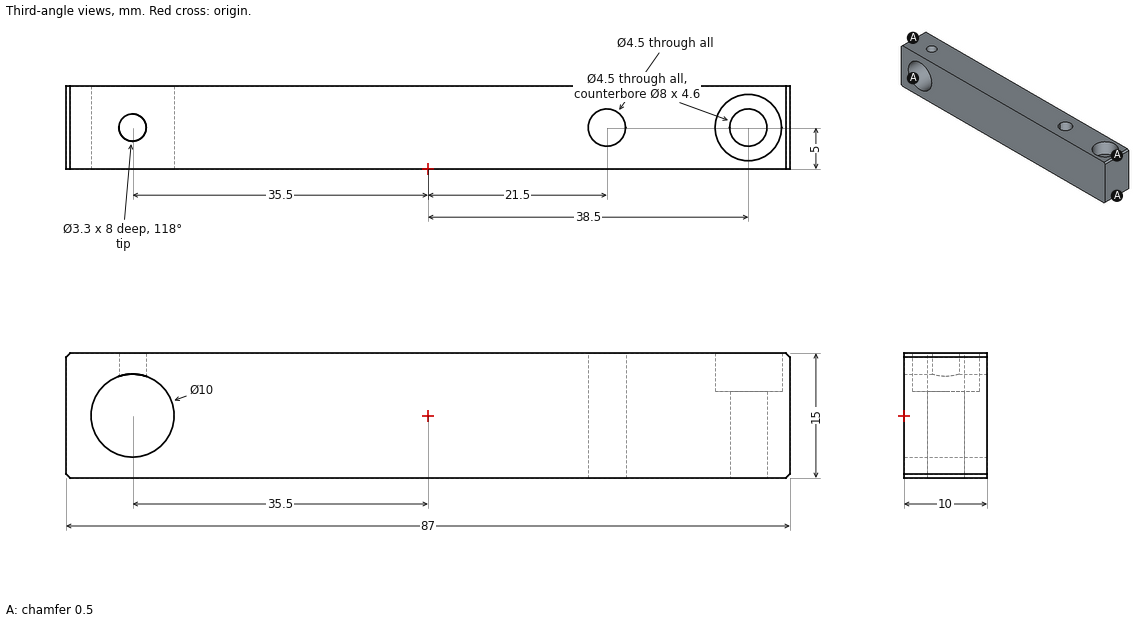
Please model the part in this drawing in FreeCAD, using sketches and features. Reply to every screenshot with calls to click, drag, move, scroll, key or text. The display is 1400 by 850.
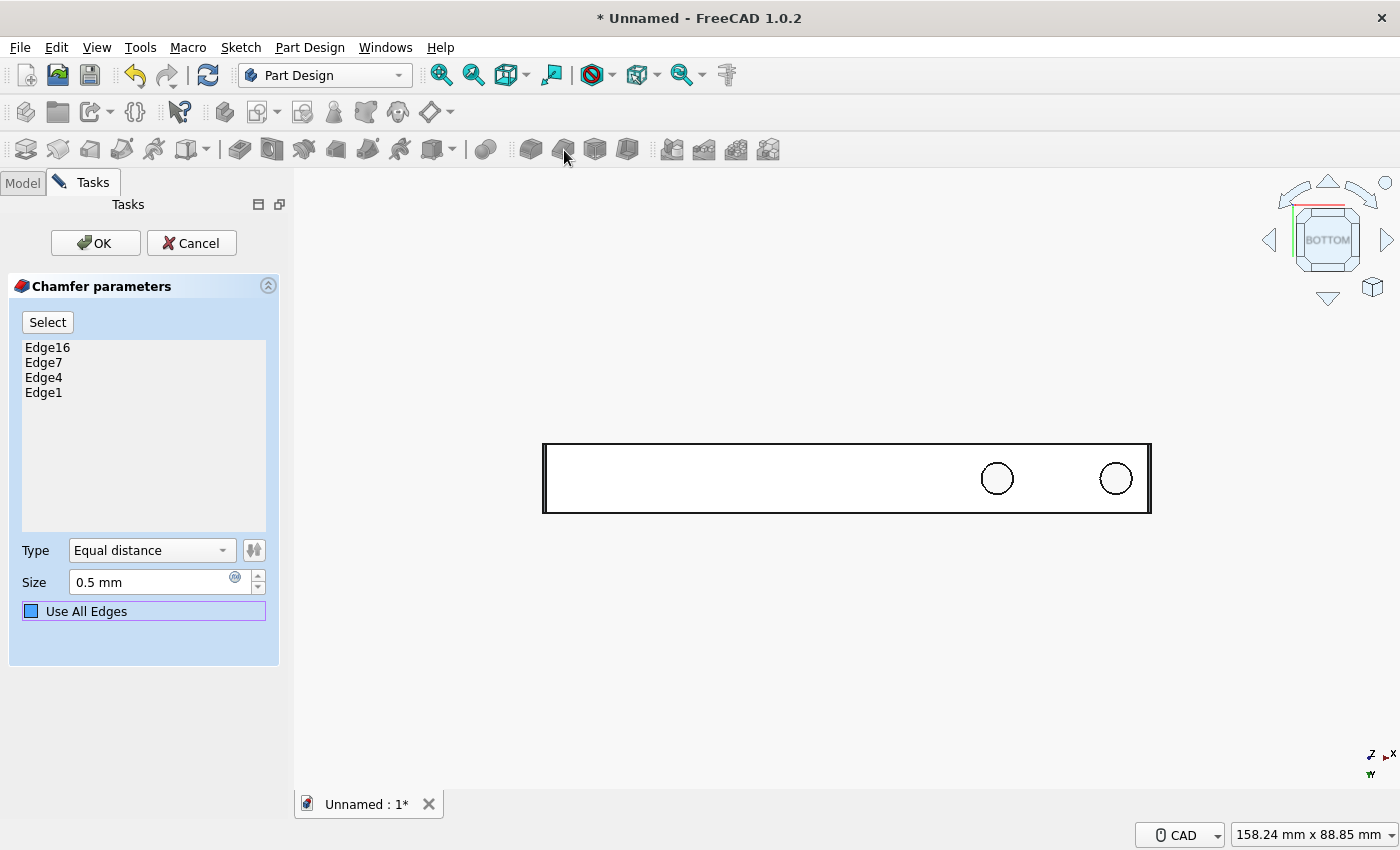
click(96, 243)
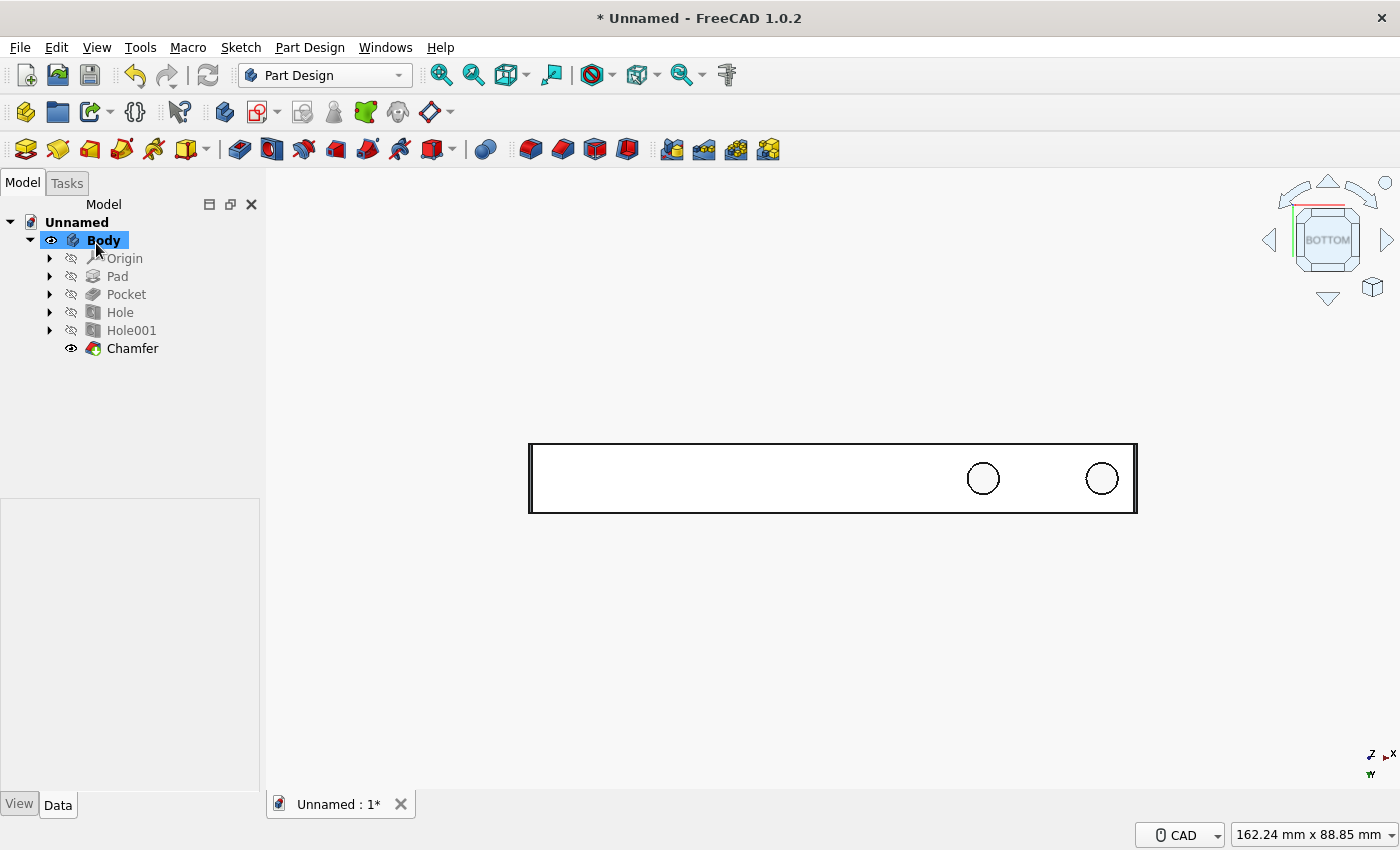
key(0)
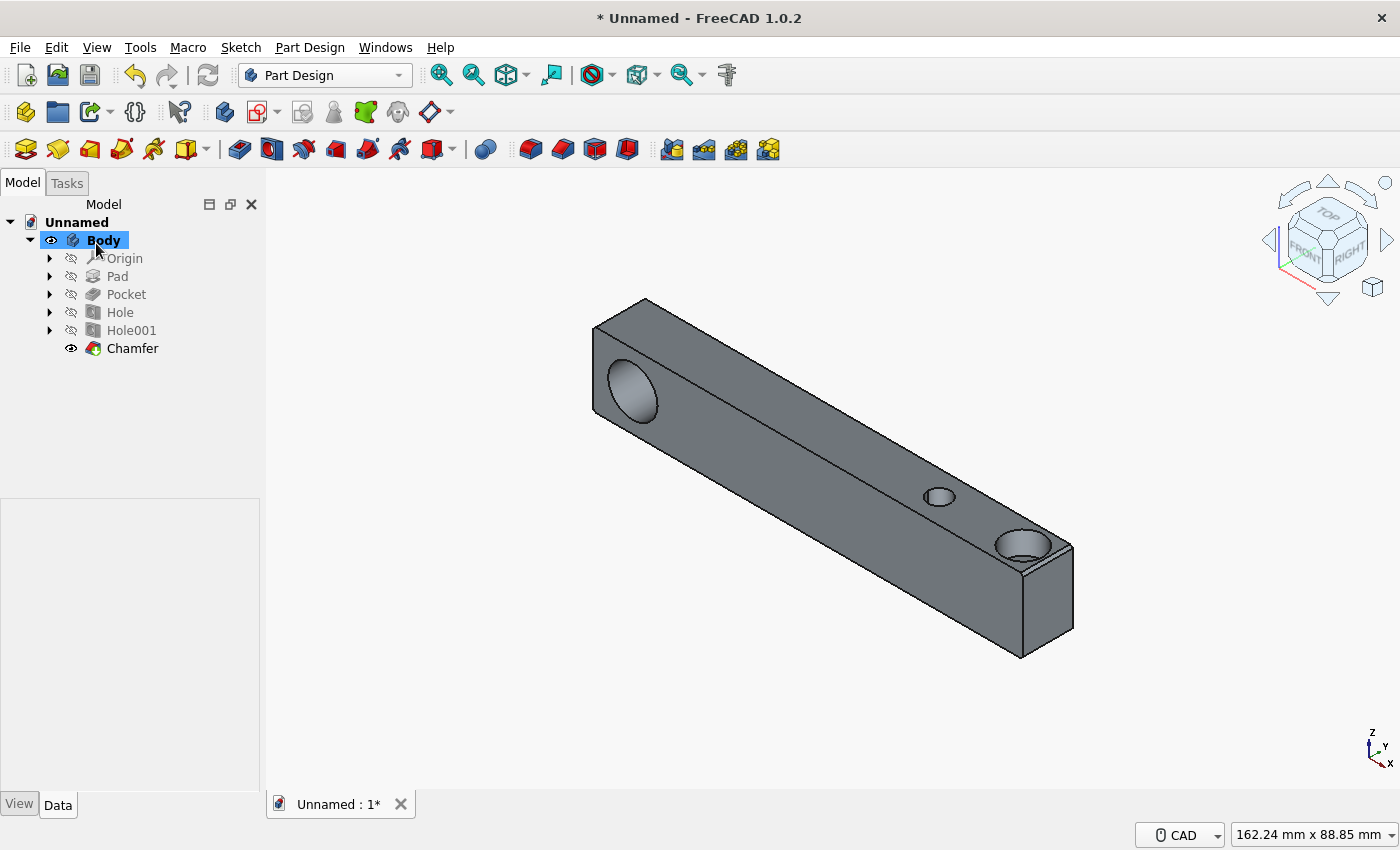
click(894, 470)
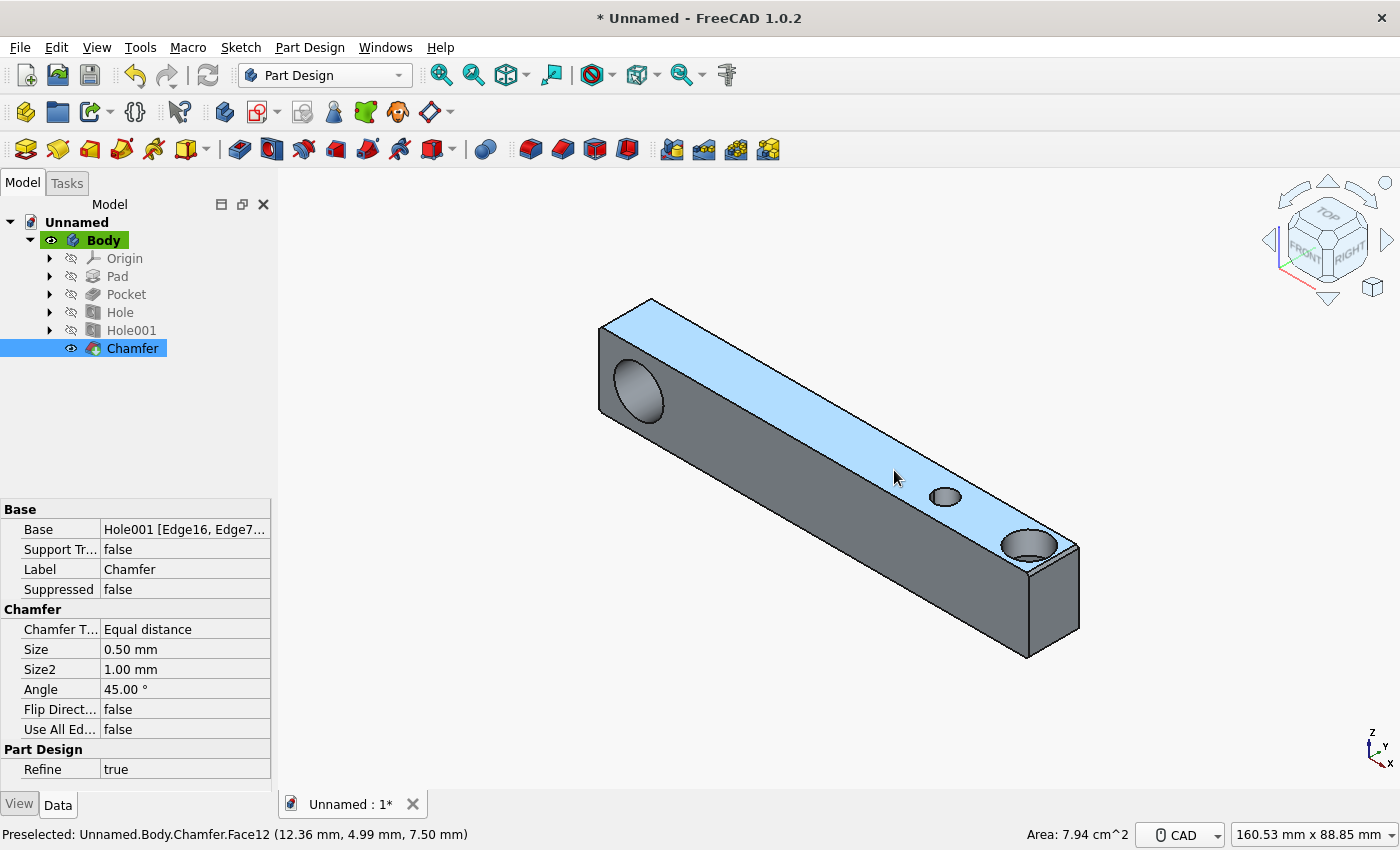
click(258, 112)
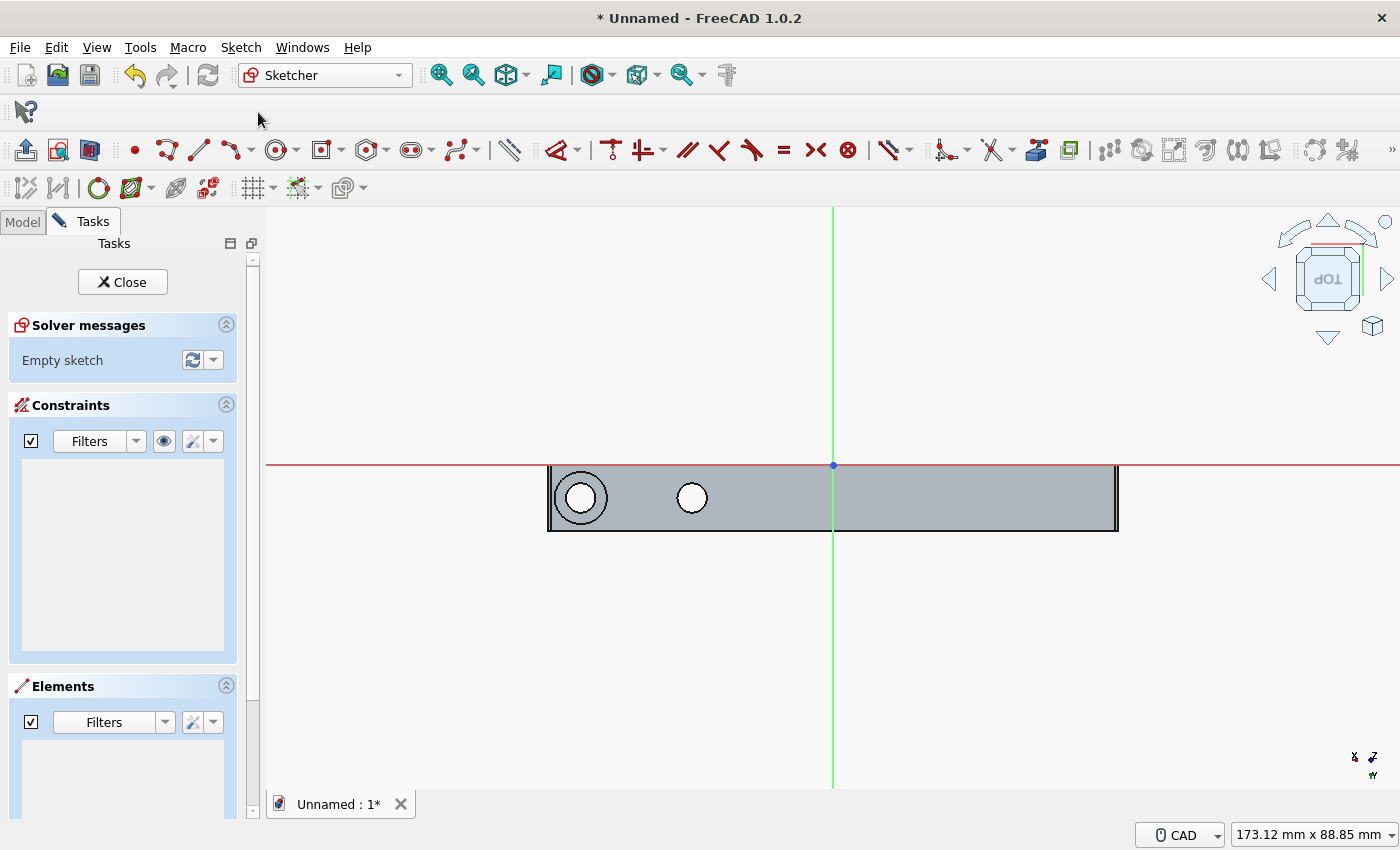
scroll(1085, 498, up, 14)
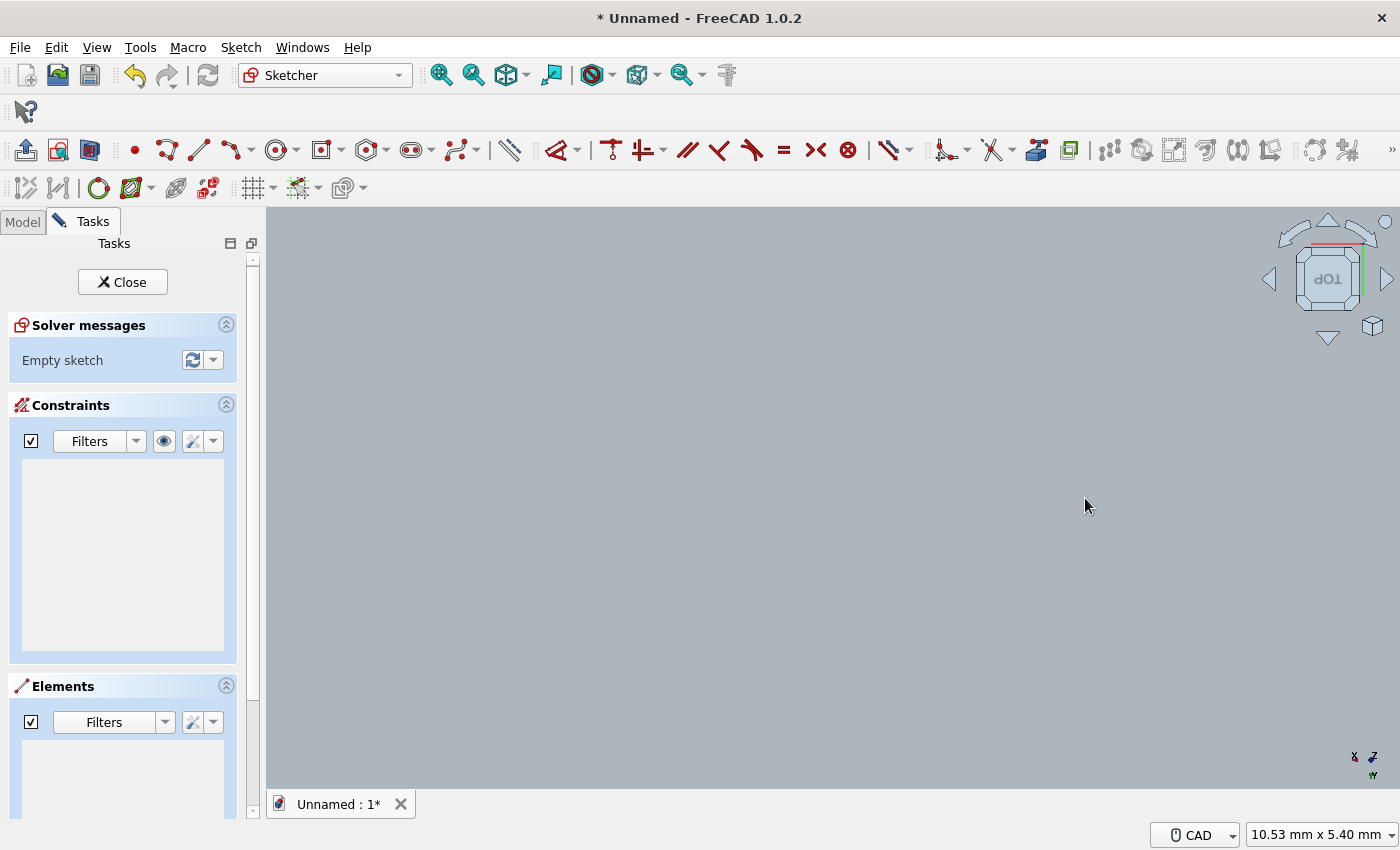
click(276, 150)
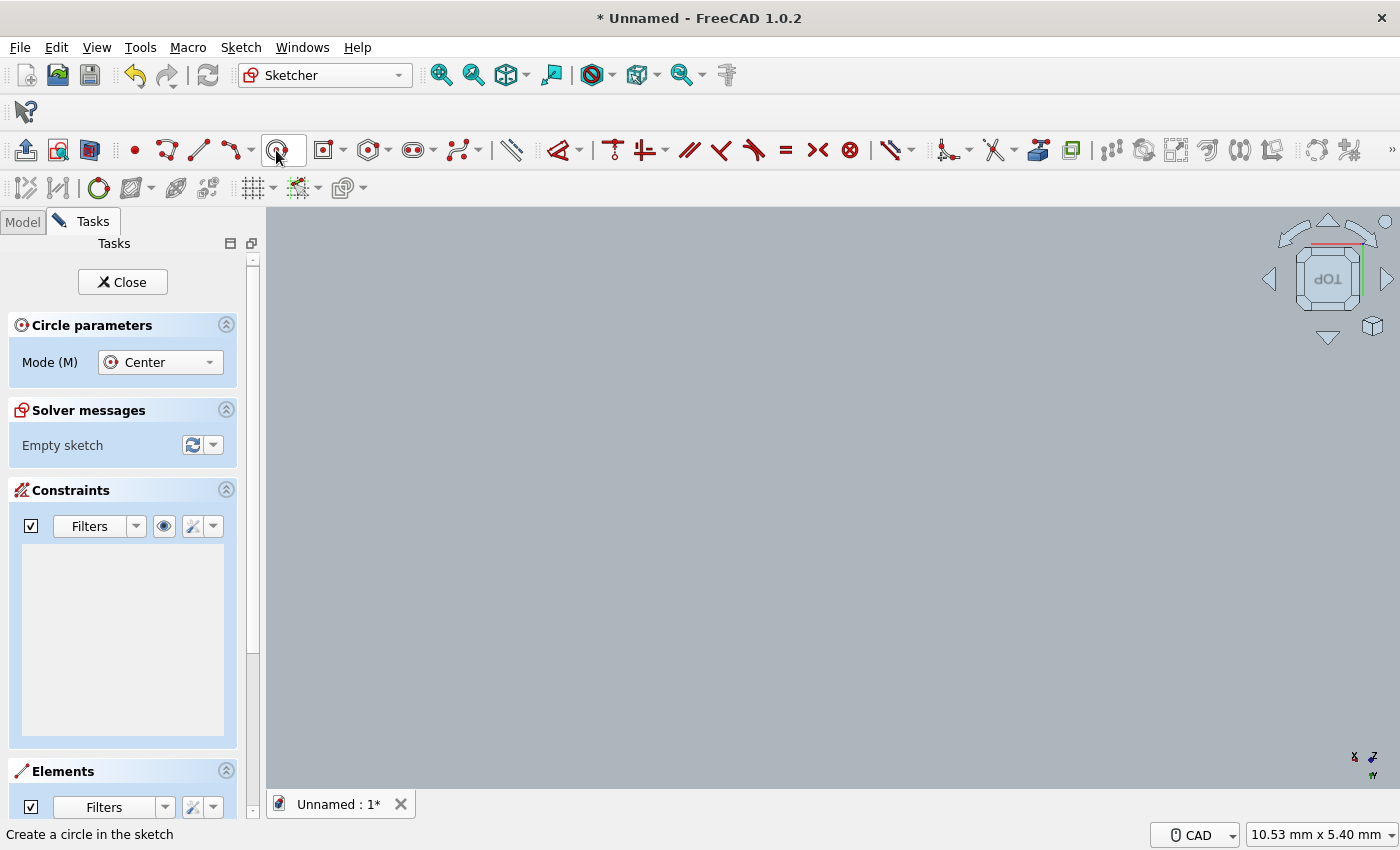
click(754, 490)
click(880, 365)
key(Escape)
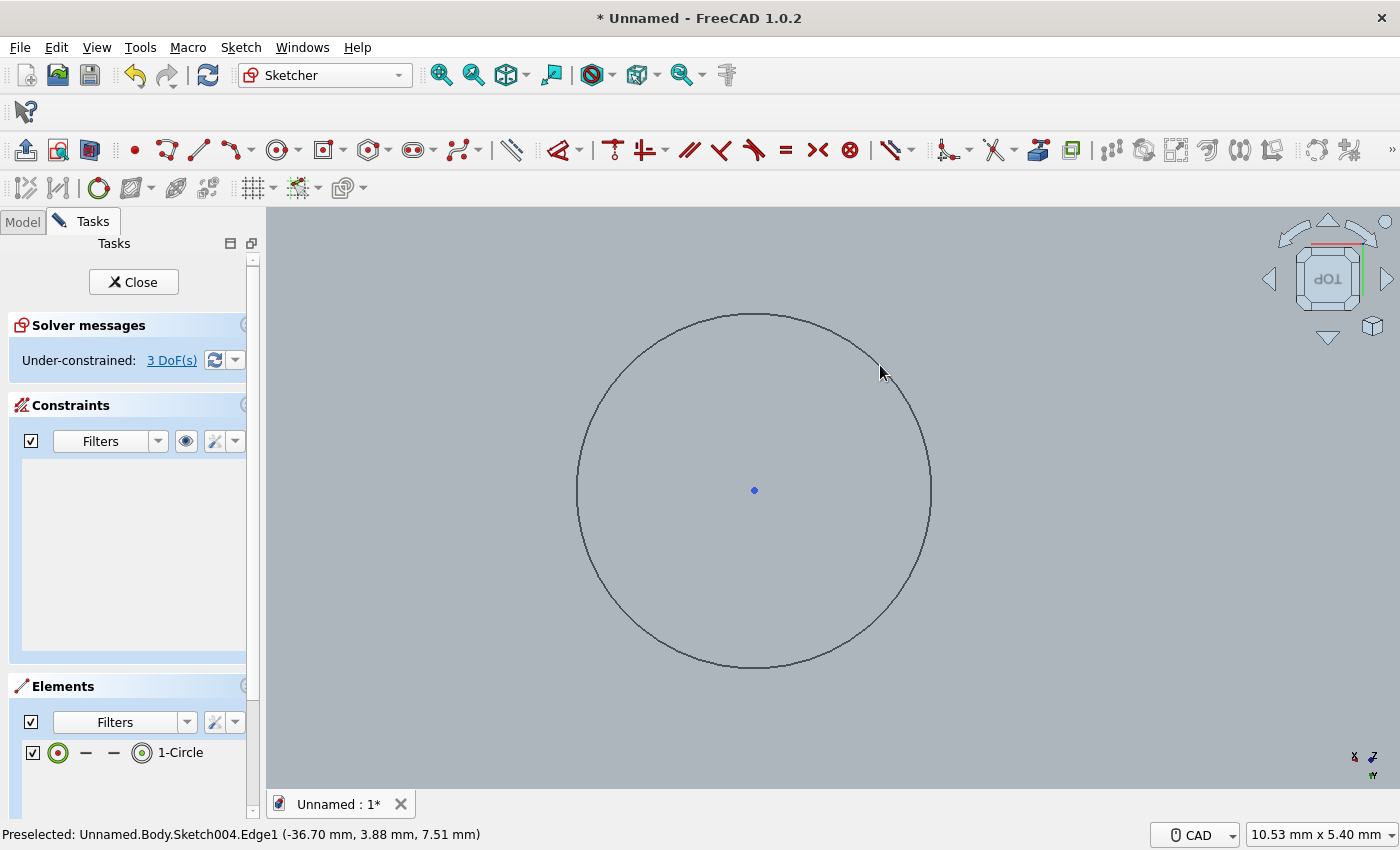
click(558, 150)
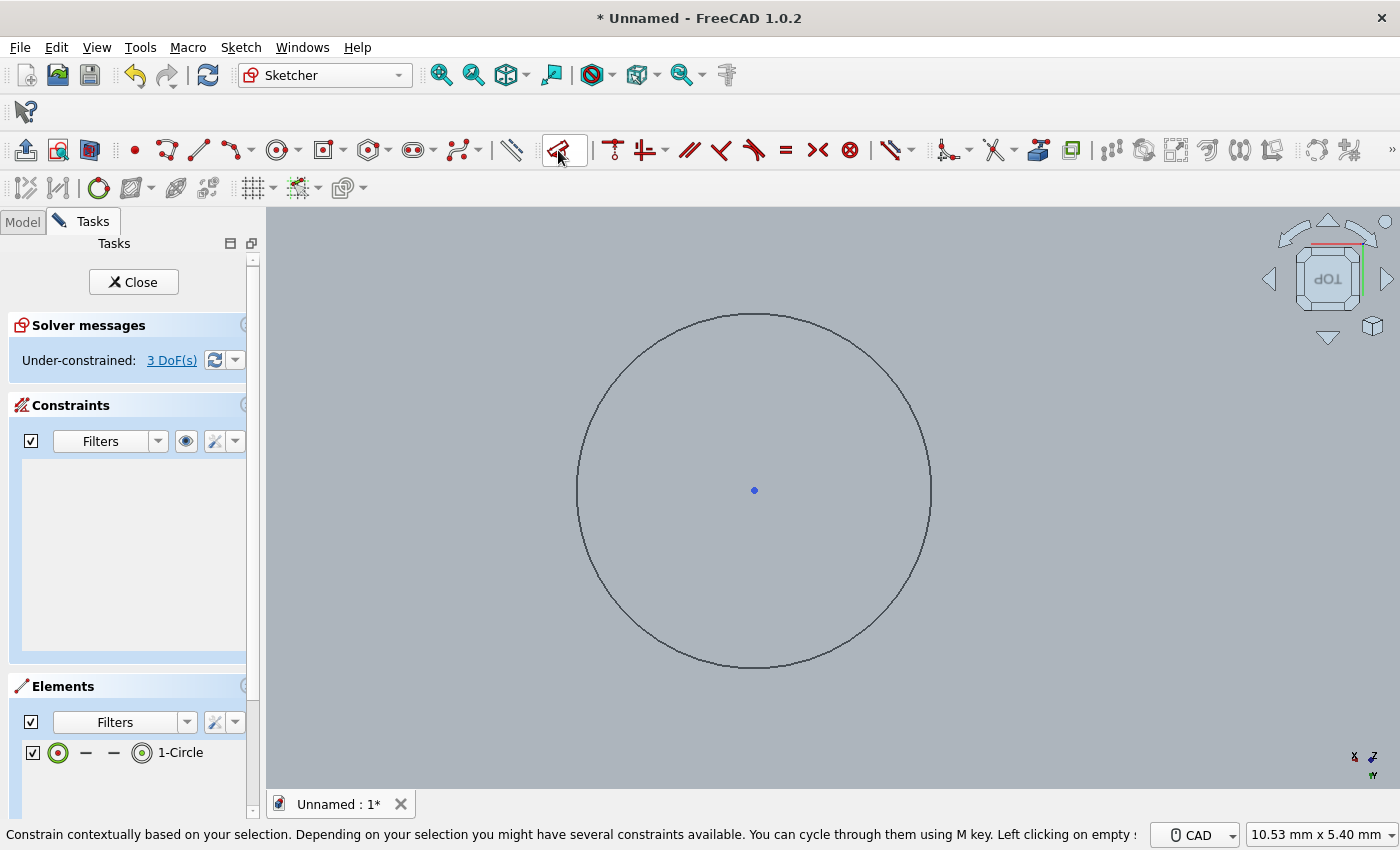
click(879, 365)
click(902, 342)